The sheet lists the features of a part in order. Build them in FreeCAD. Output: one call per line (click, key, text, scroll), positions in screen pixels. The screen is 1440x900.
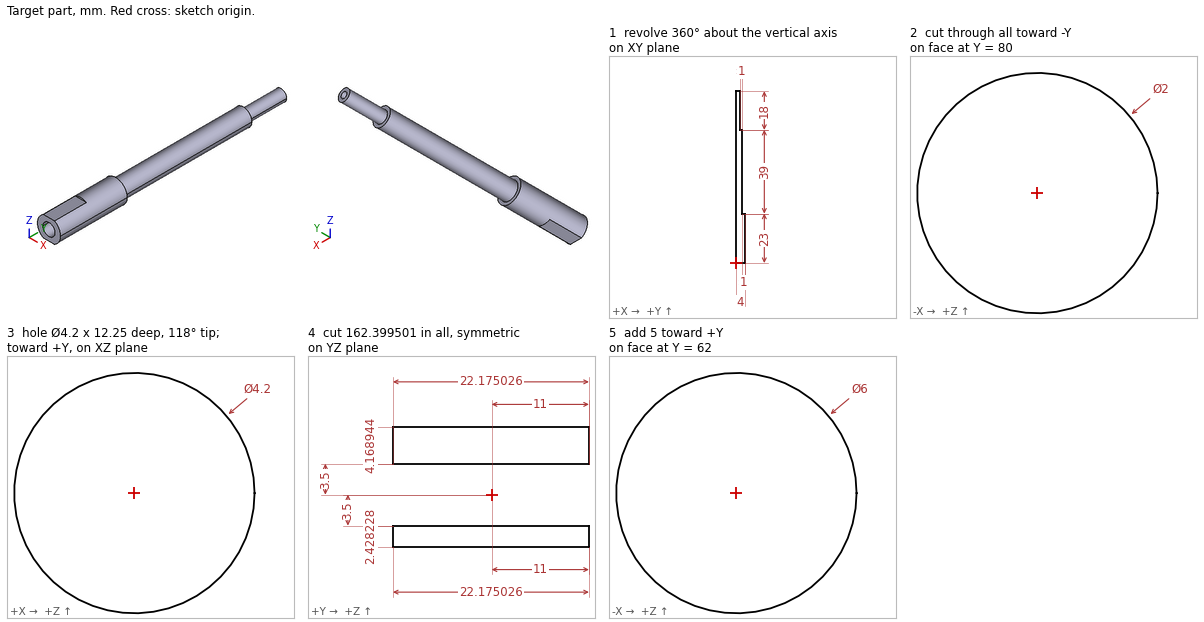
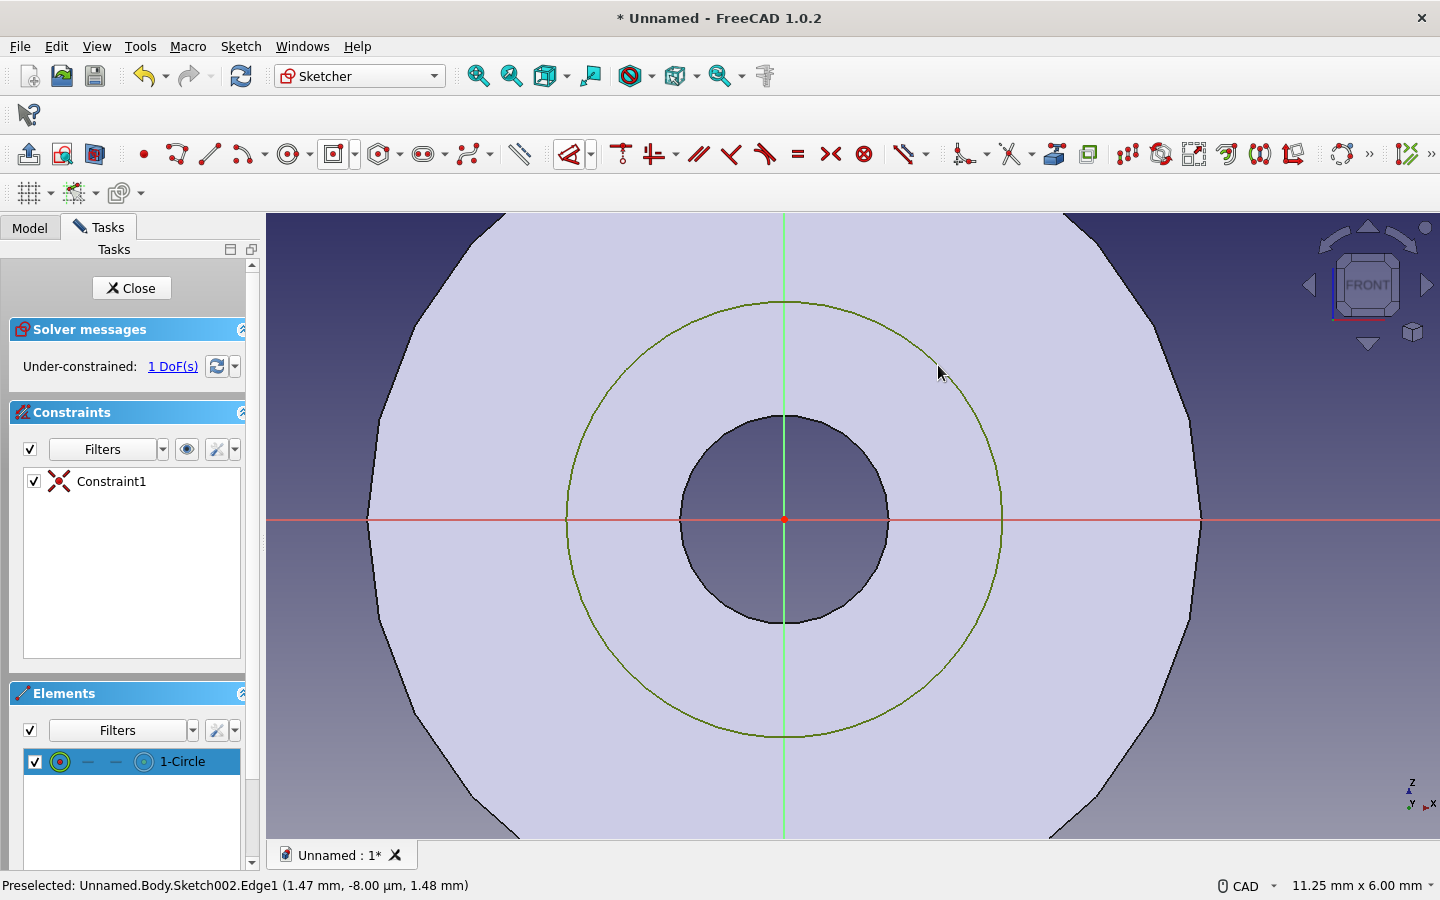
key(k)
key(o)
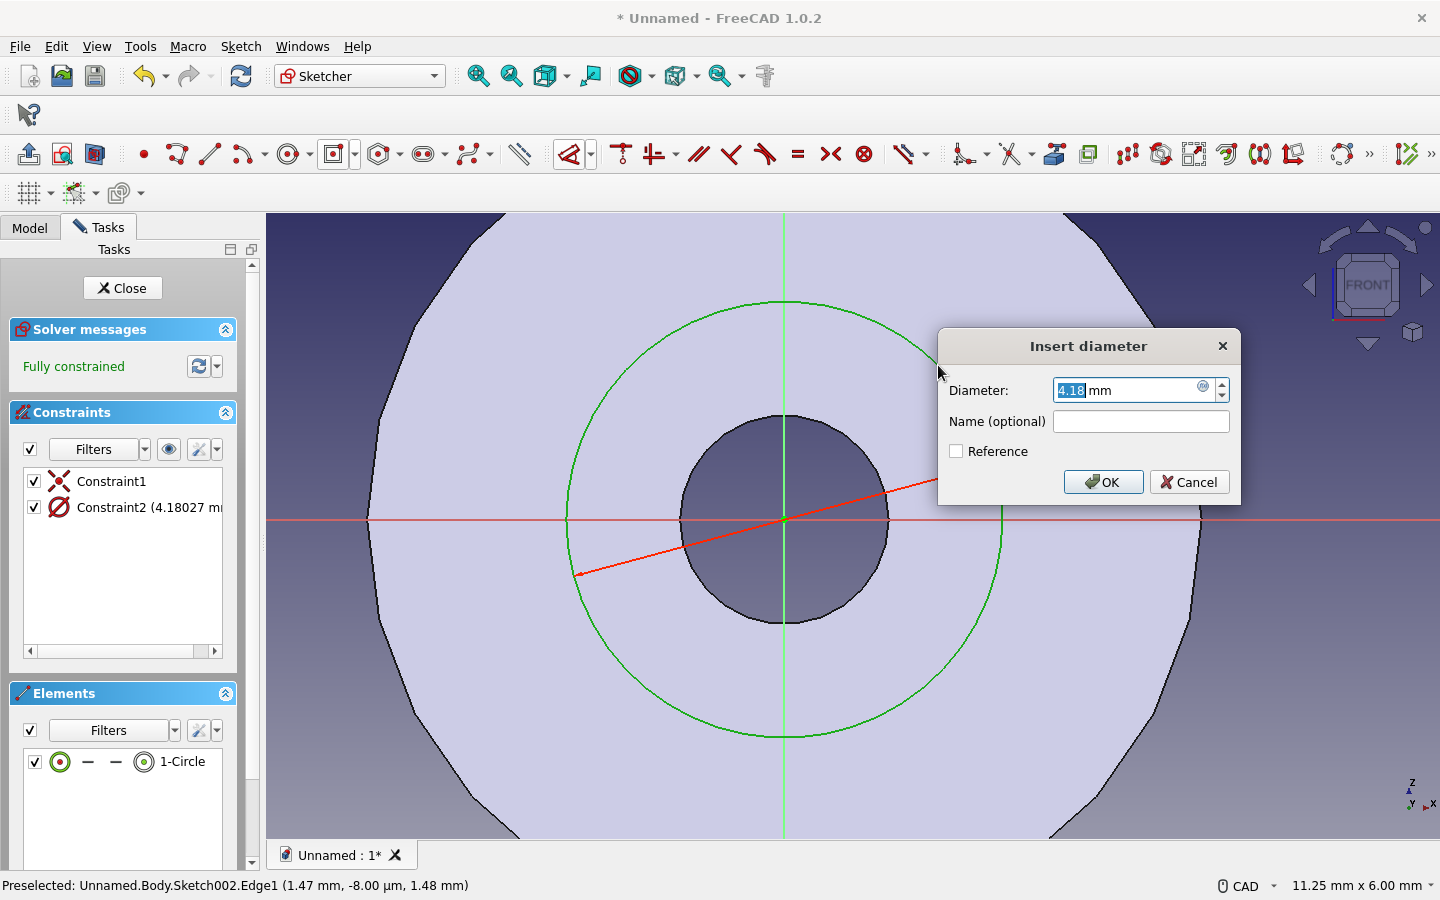
text(4.2)
key(Return)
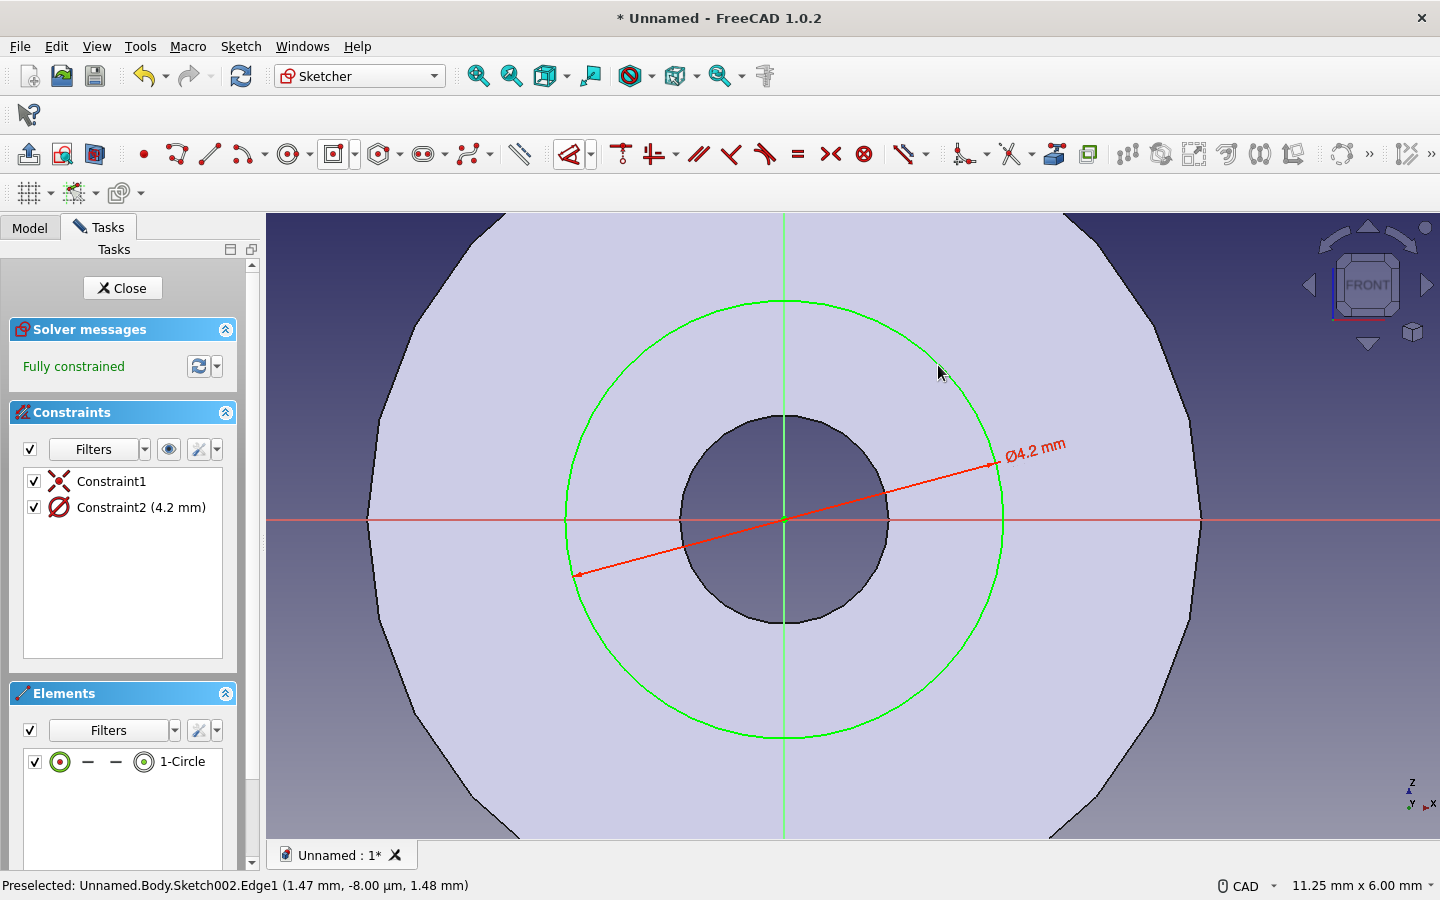
click(123, 288)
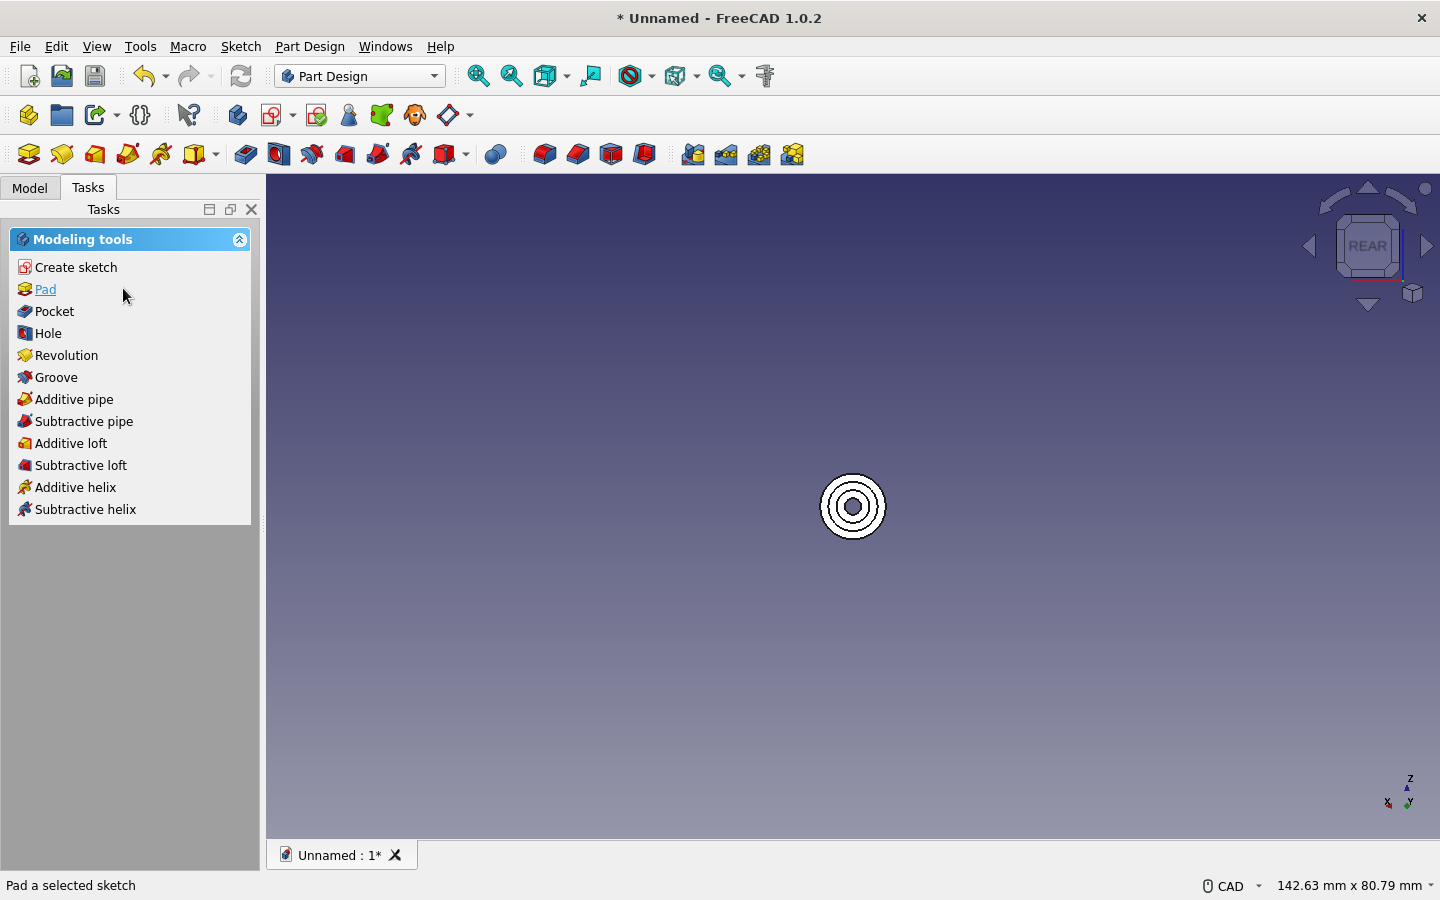
click(279, 154)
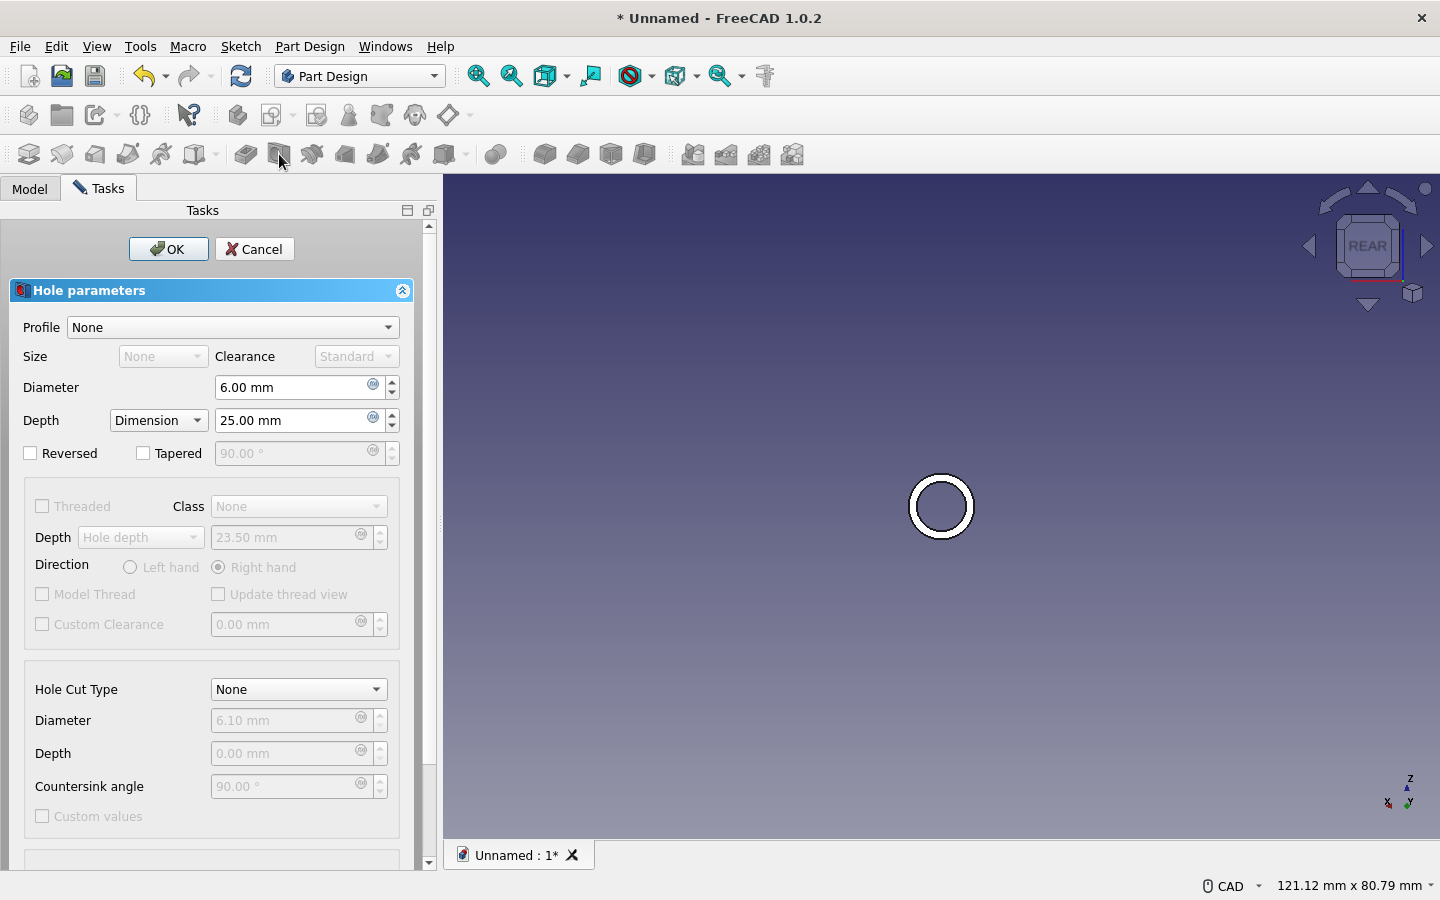
triple_click(300, 388)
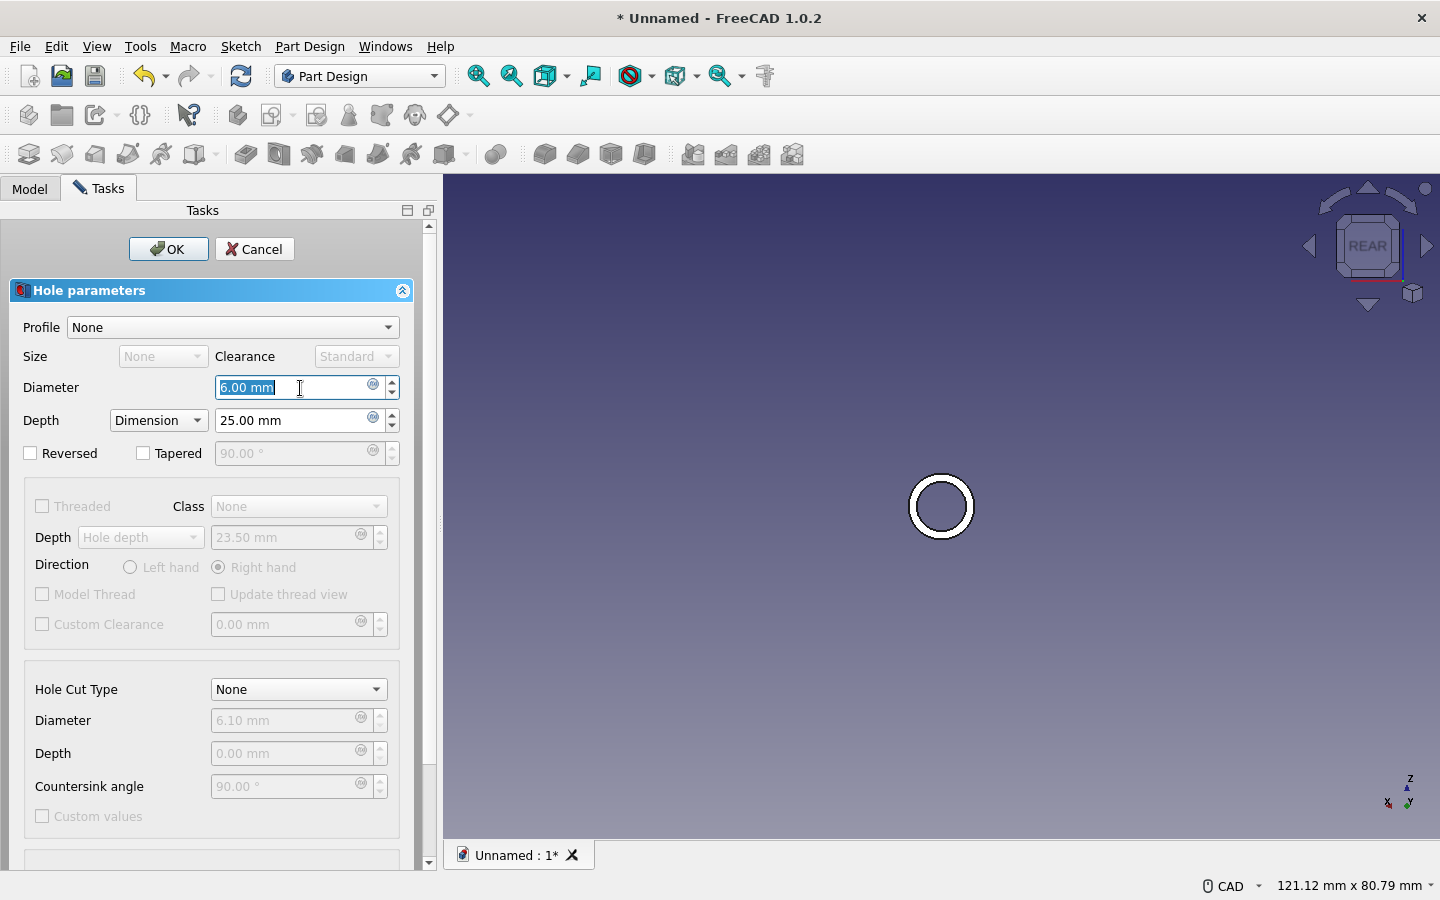
text(4.2)
key(Tab)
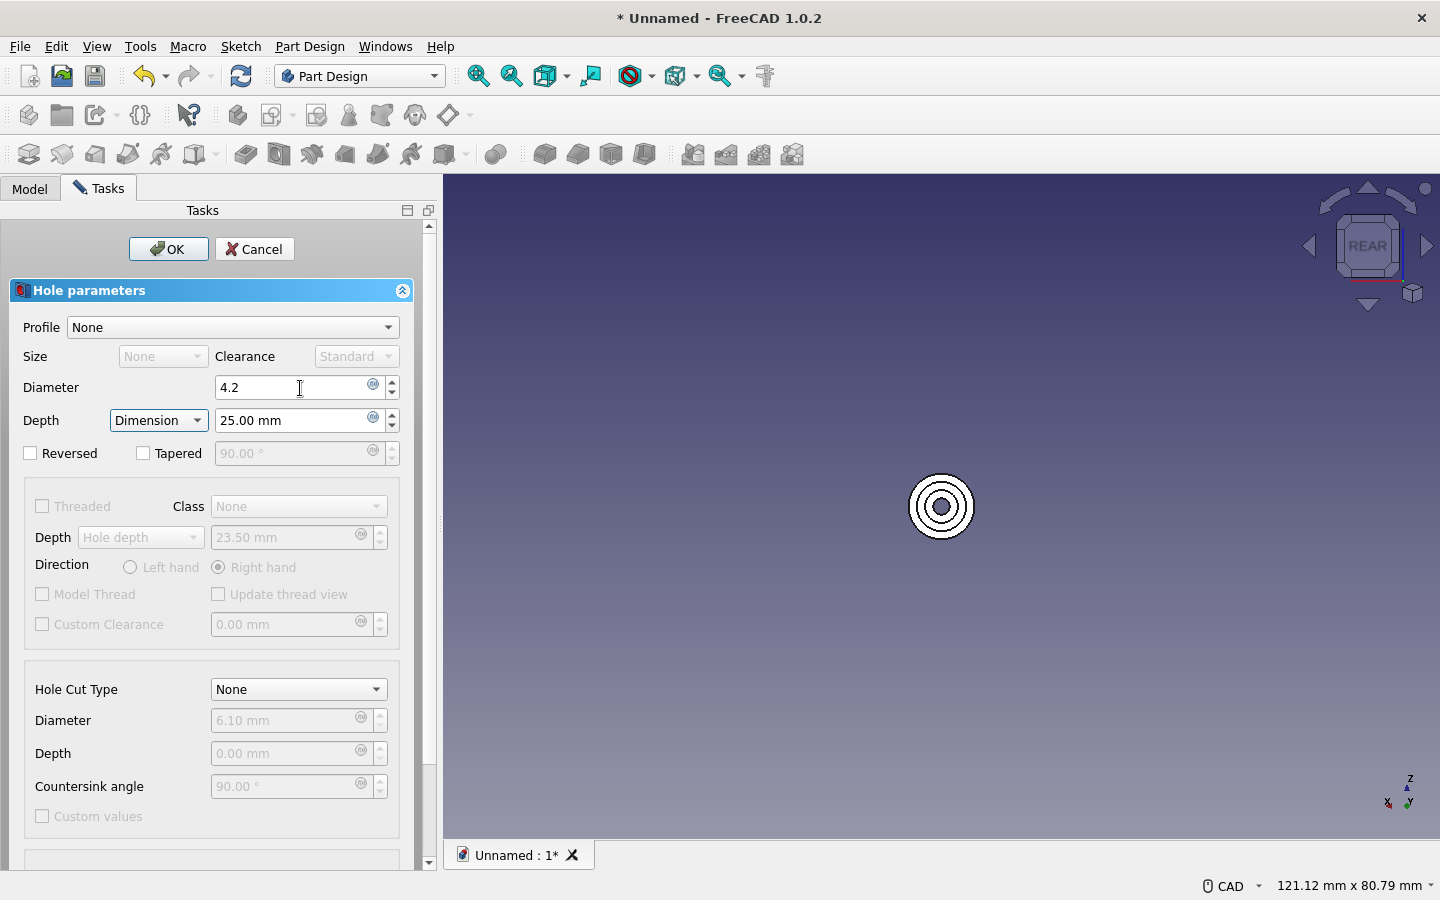
triple_click(300, 420)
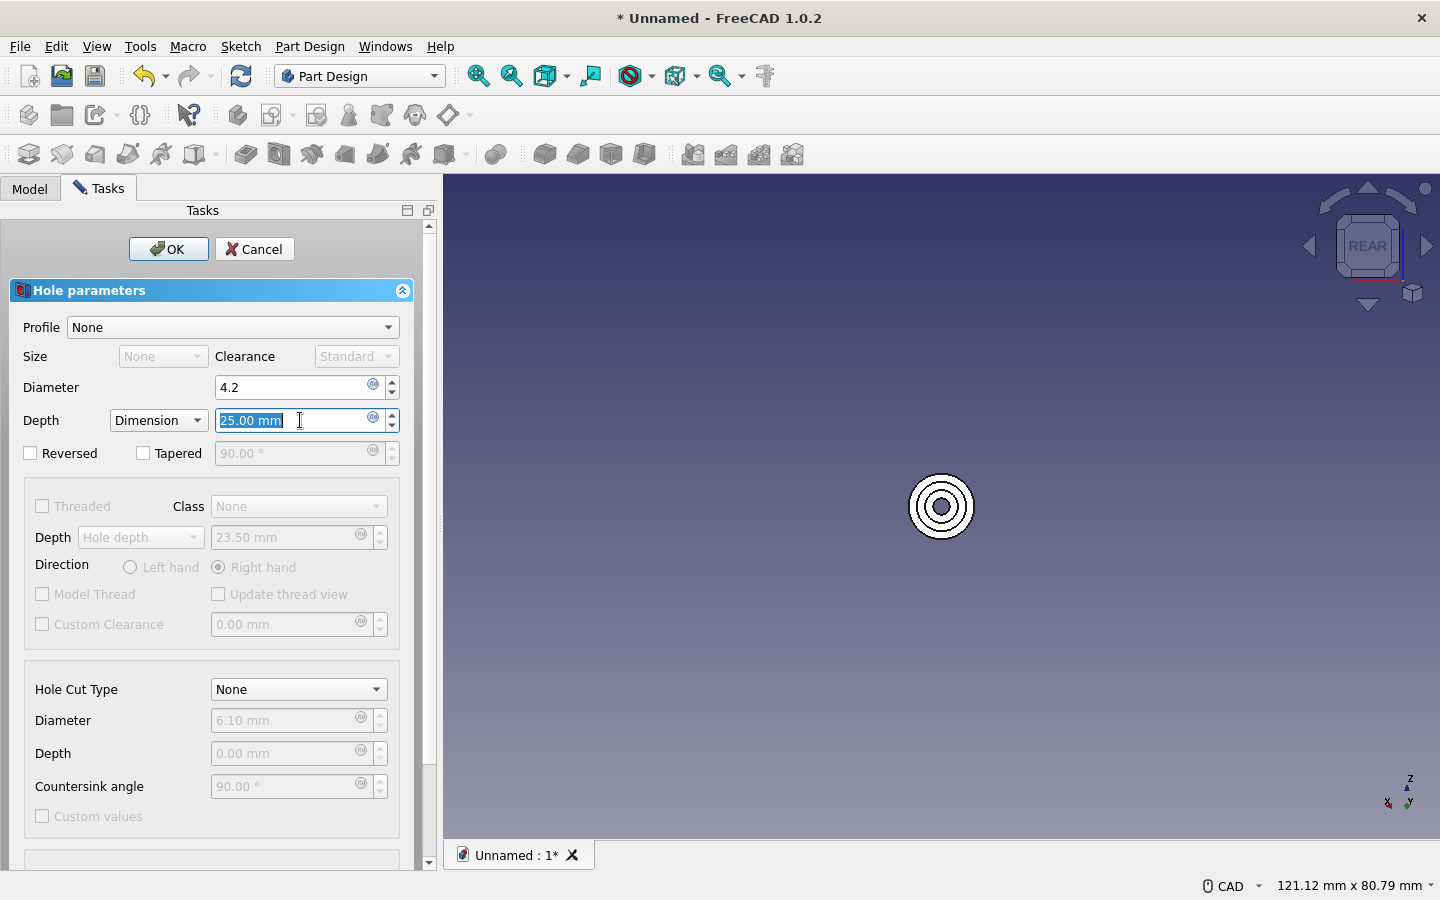
text(12.25)
key(Tab)